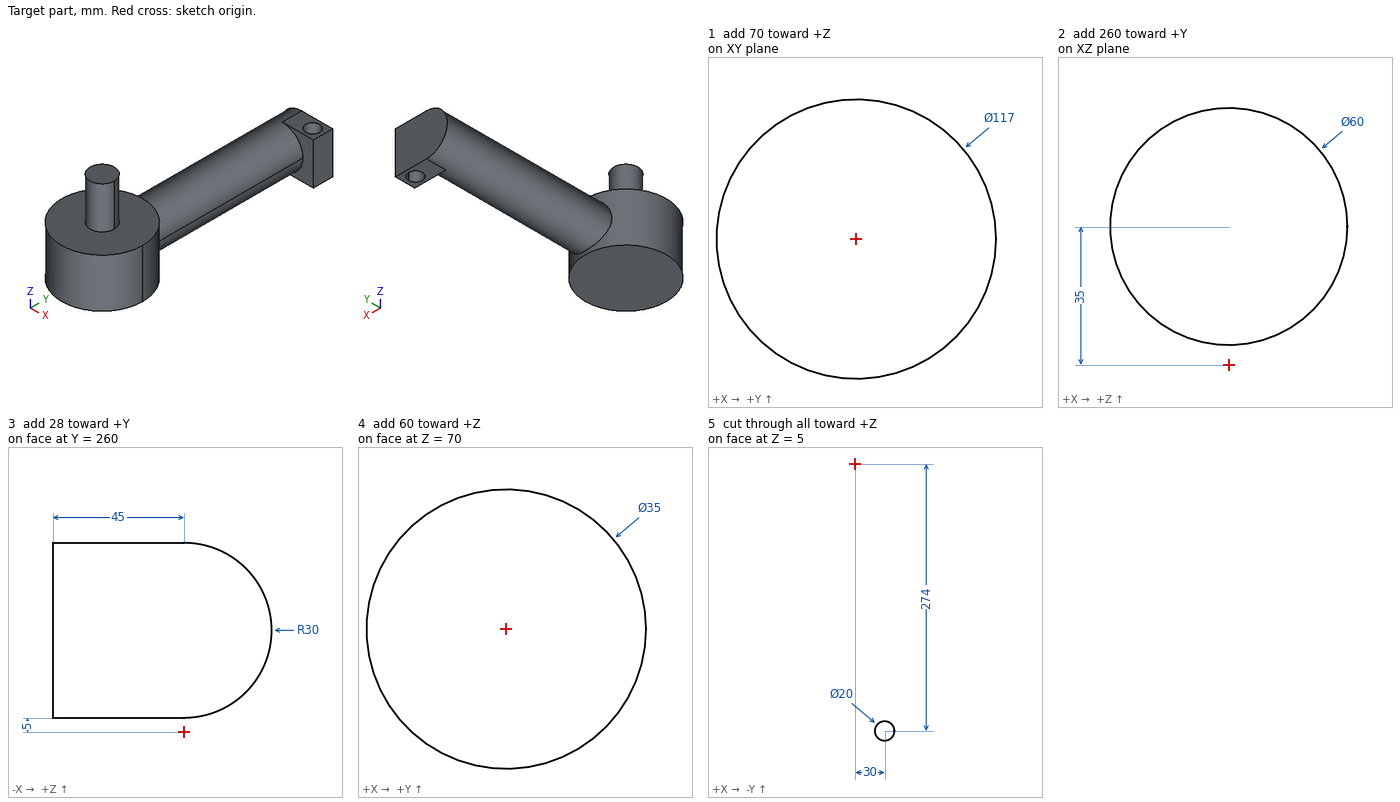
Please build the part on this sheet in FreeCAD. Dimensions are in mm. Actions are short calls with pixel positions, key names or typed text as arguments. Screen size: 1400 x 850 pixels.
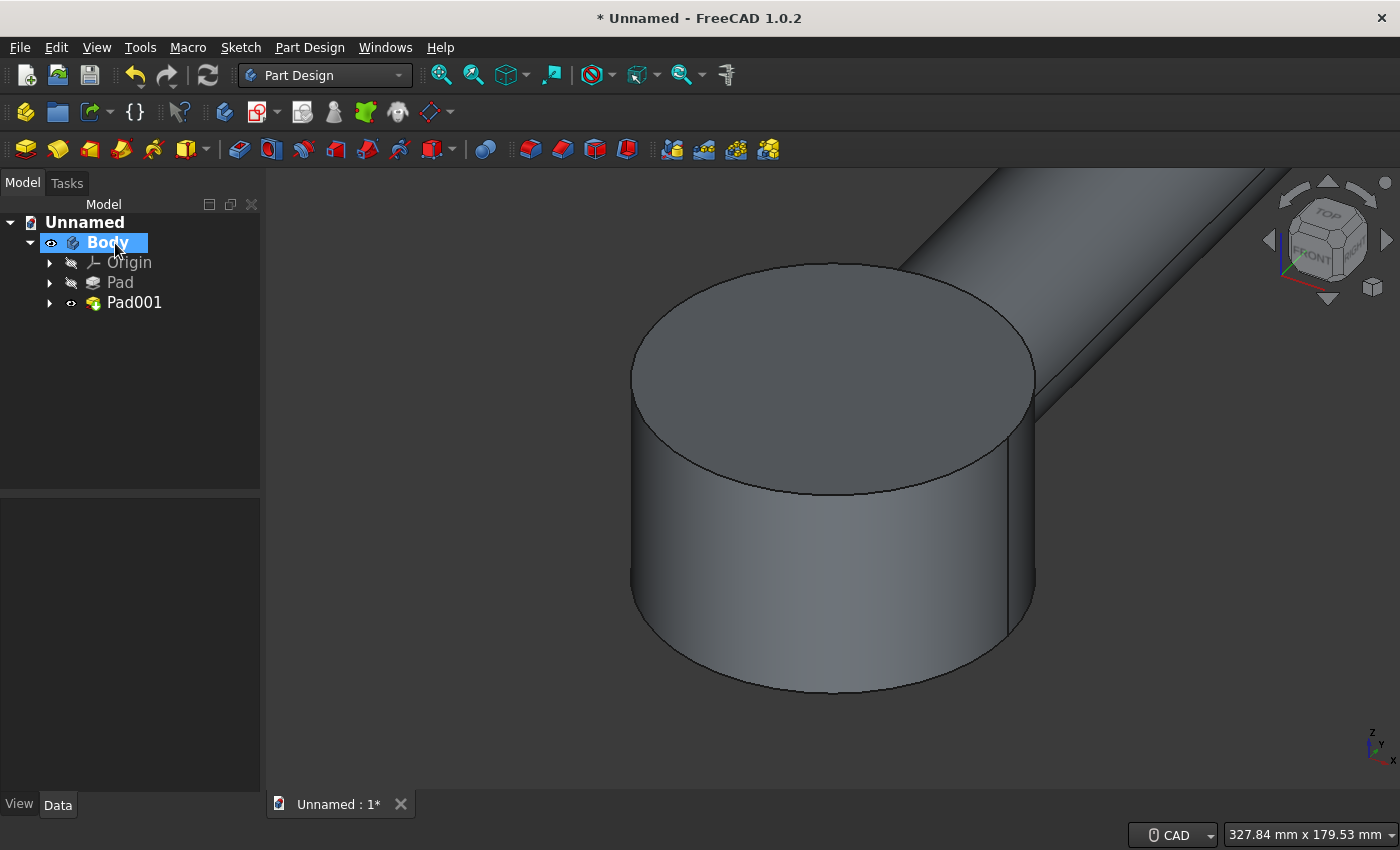
key(v)
key(f)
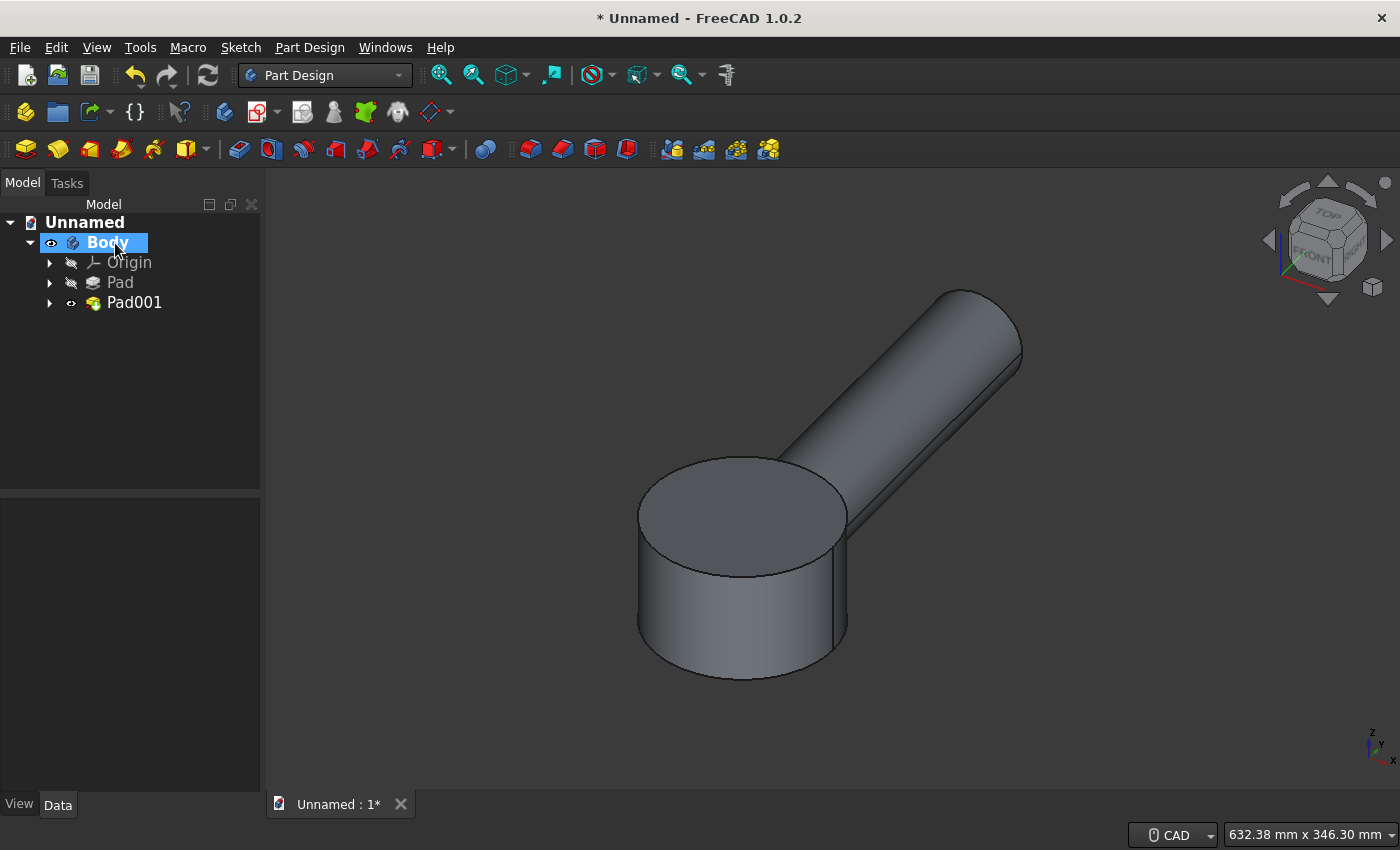
key(4)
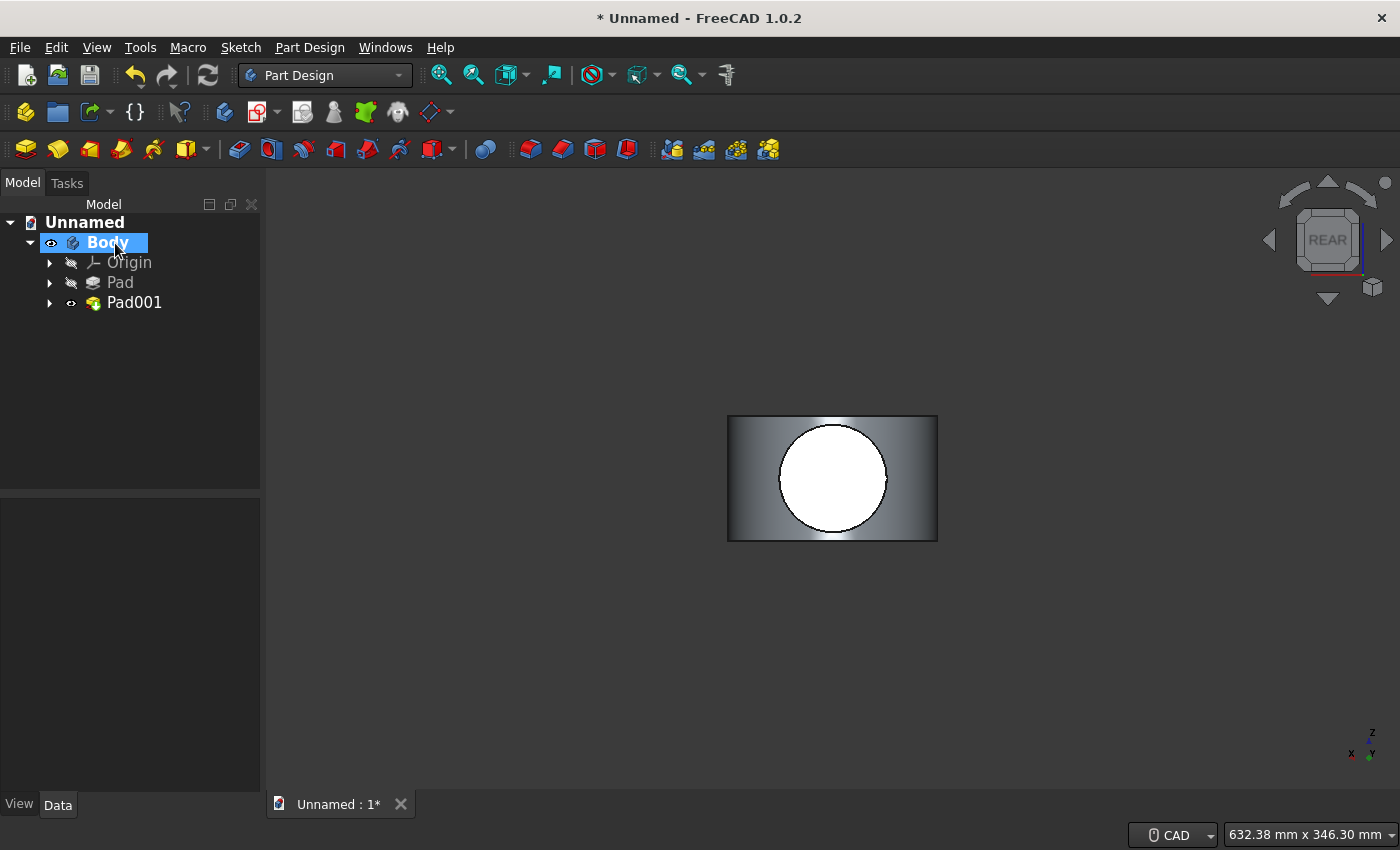
key(v)
key(f)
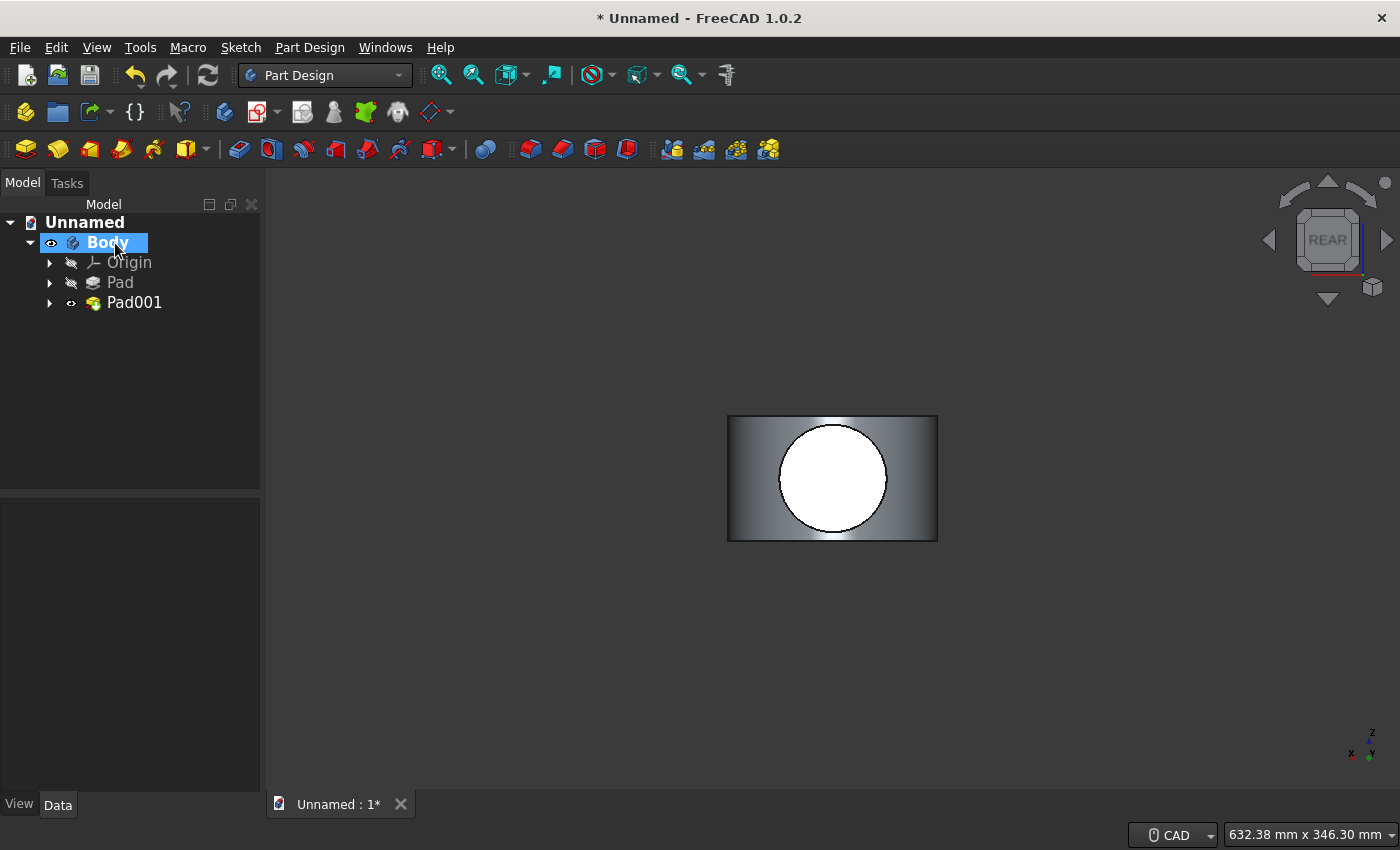
click(833, 478)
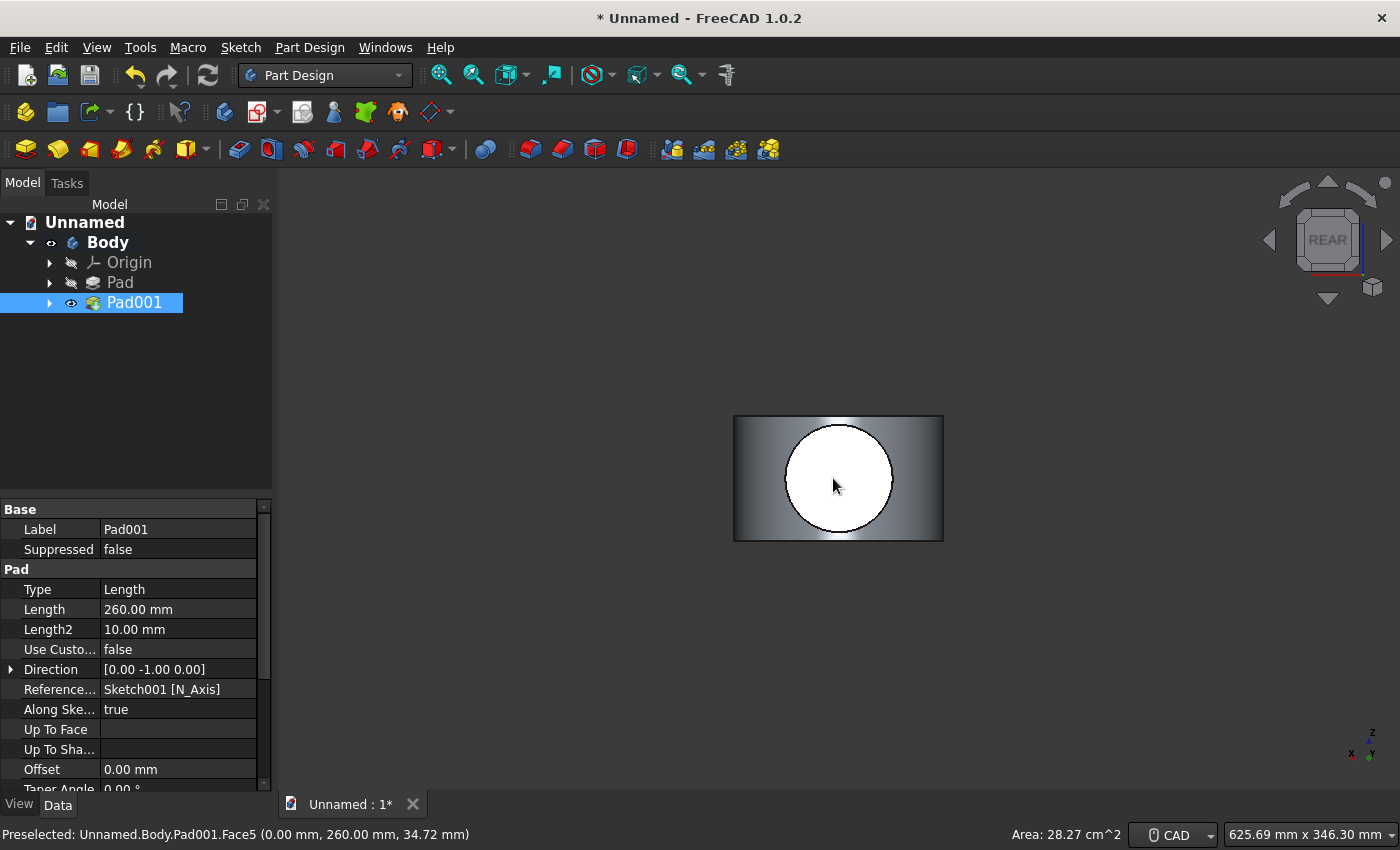
click(258, 112)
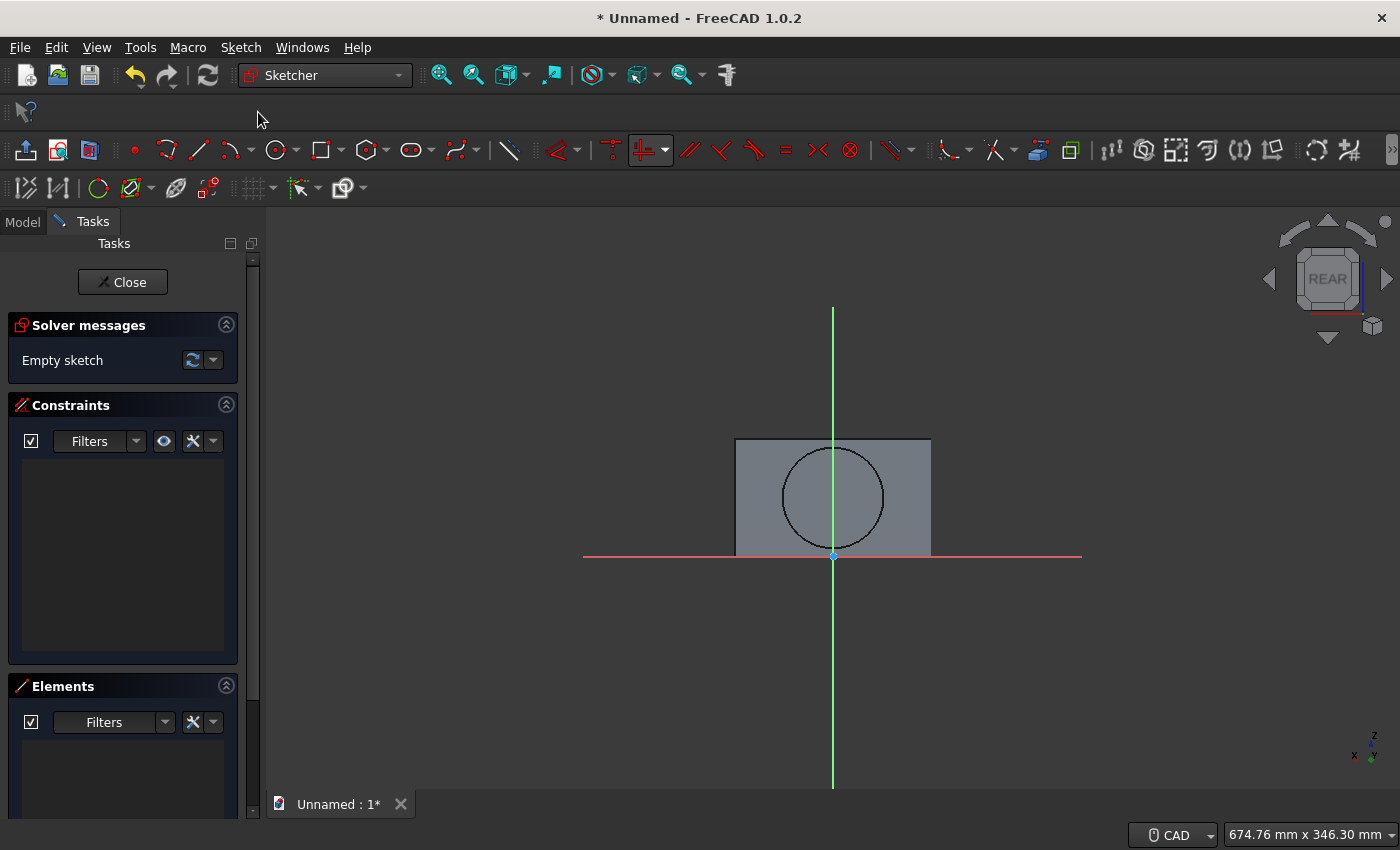
scroll(844, 504, up, 6)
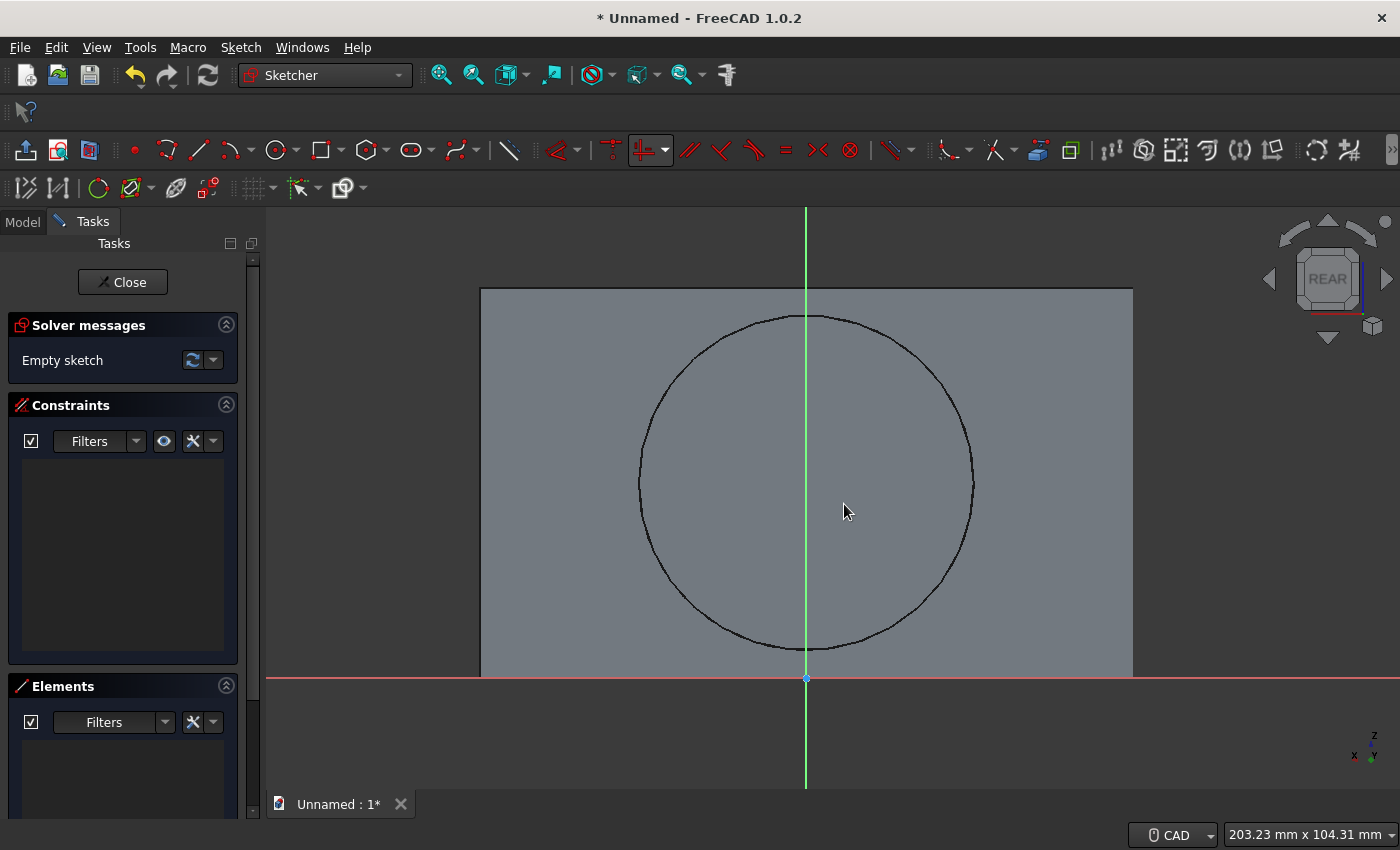
key(g)
key(m)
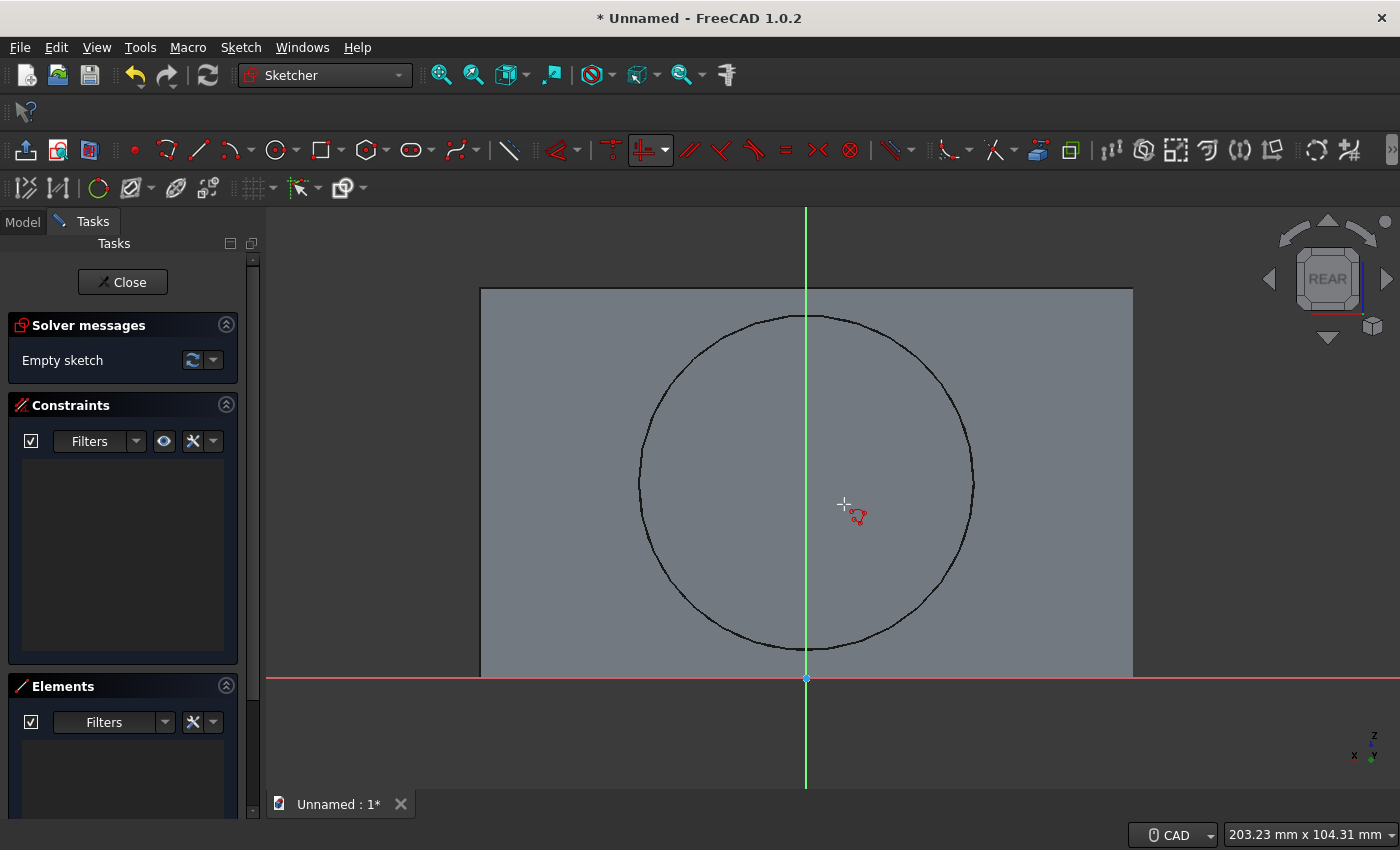
click(806, 315)
click(555, 315)
click(555, 650)
click(806, 650)
right_click(806, 650)